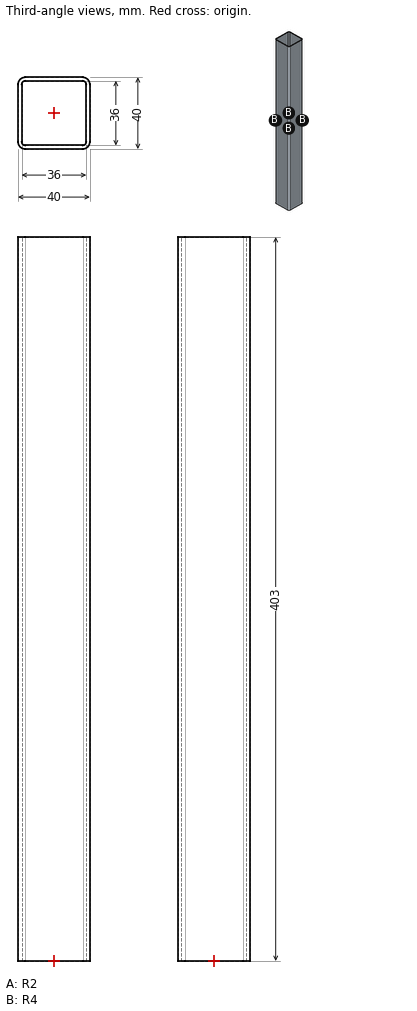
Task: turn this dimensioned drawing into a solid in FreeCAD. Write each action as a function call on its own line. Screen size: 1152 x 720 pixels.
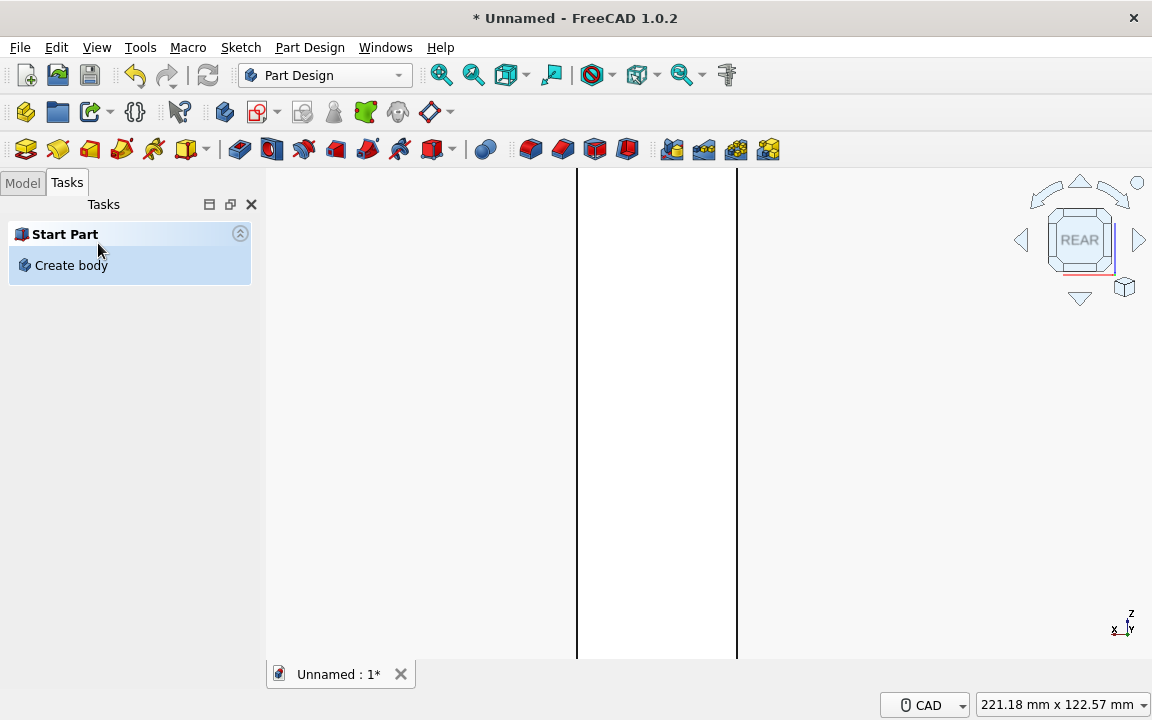
key(v)
key(f)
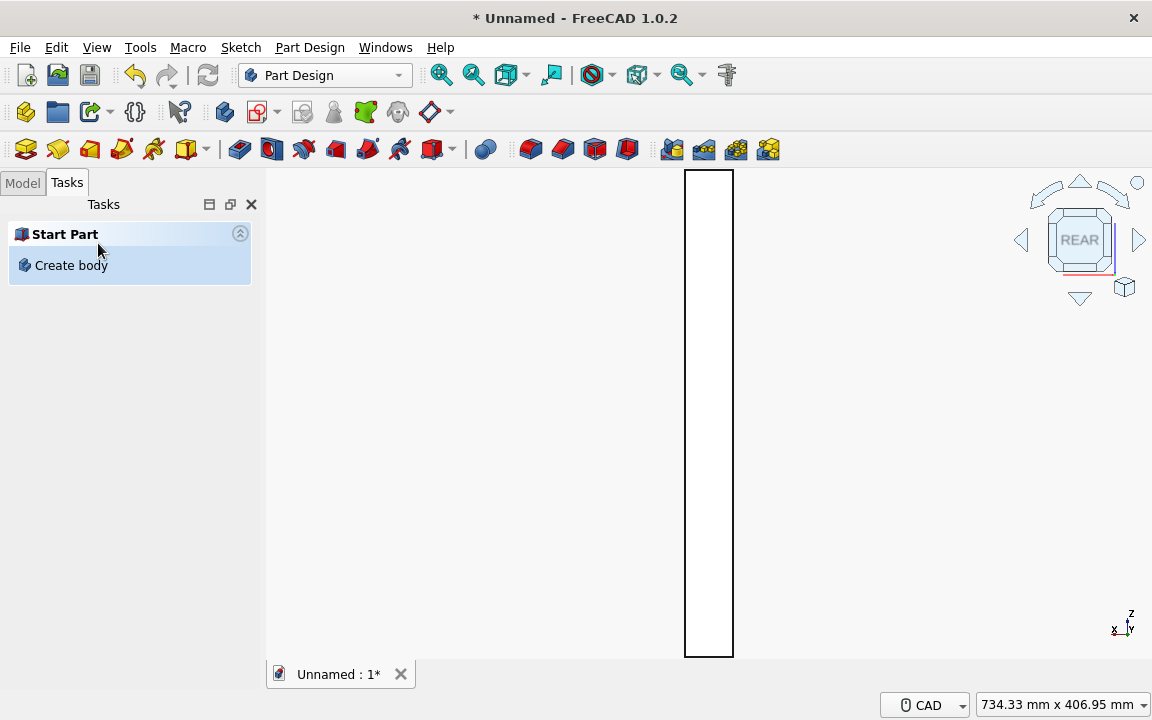
click(733, 413)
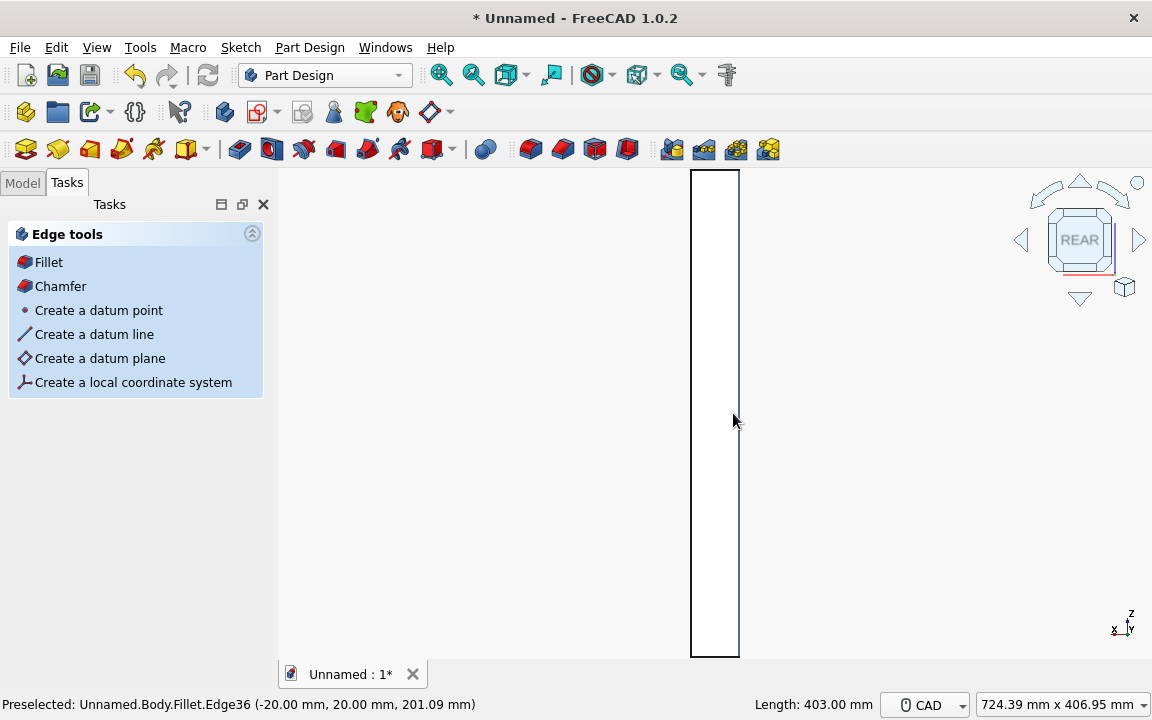
click(691, 413, ctrl)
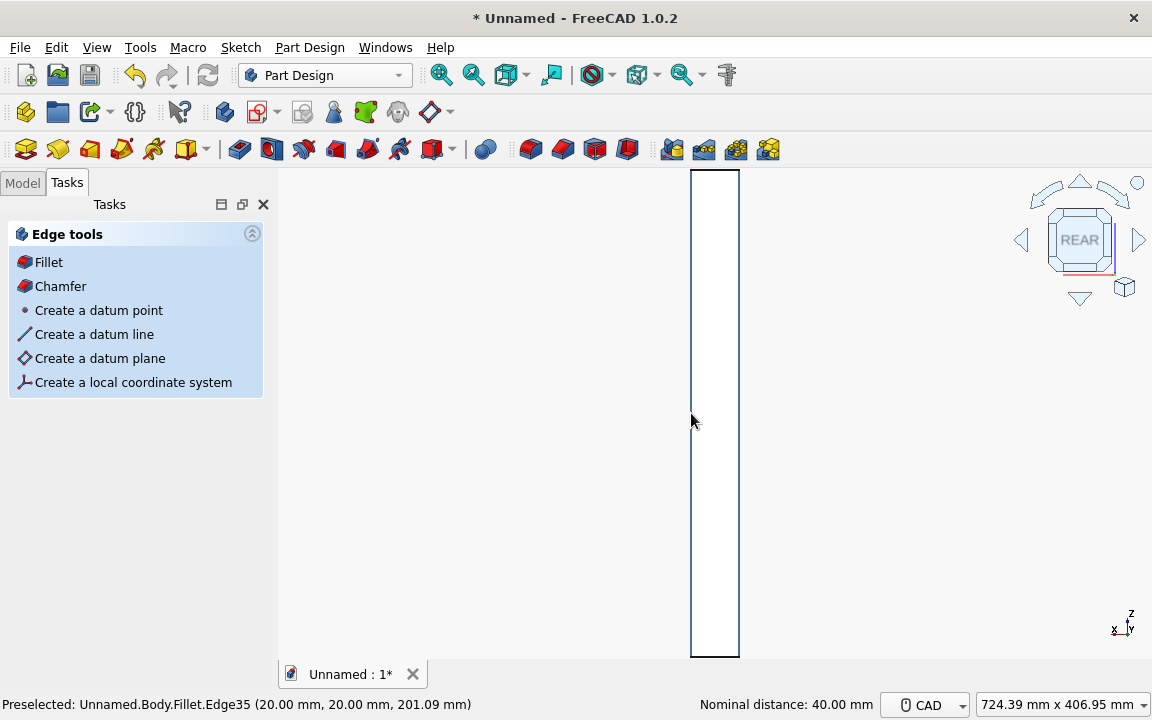
key(0)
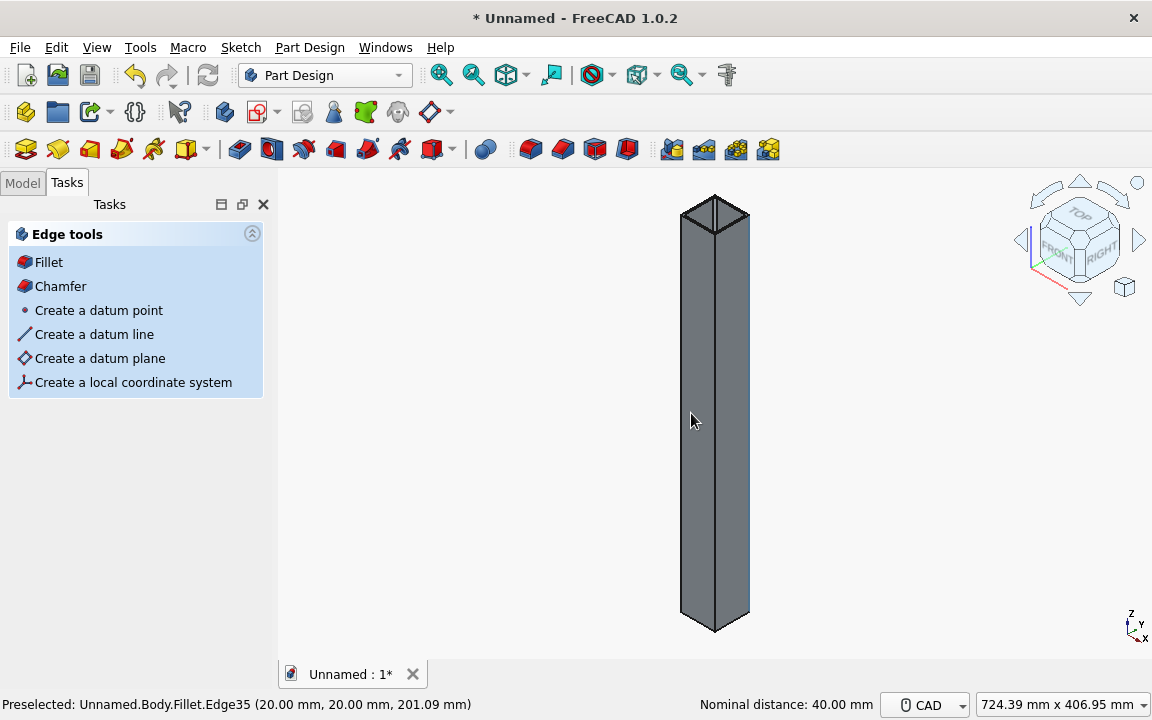
click(715, 432, ctrl)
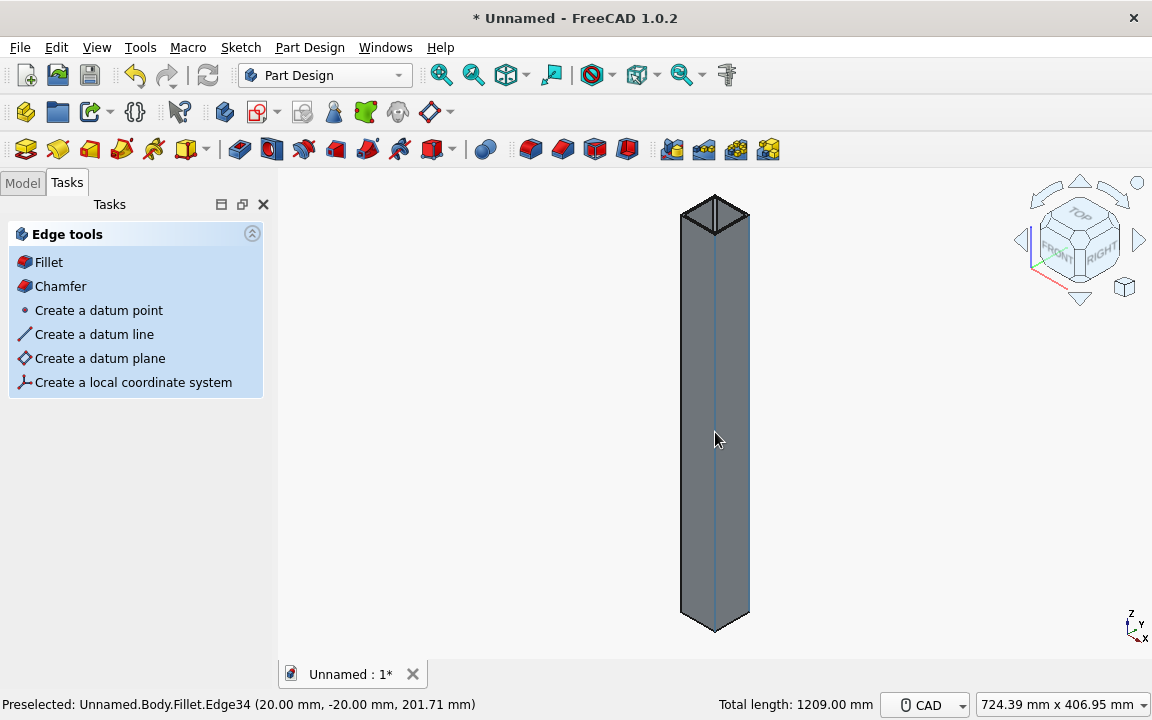
key(2)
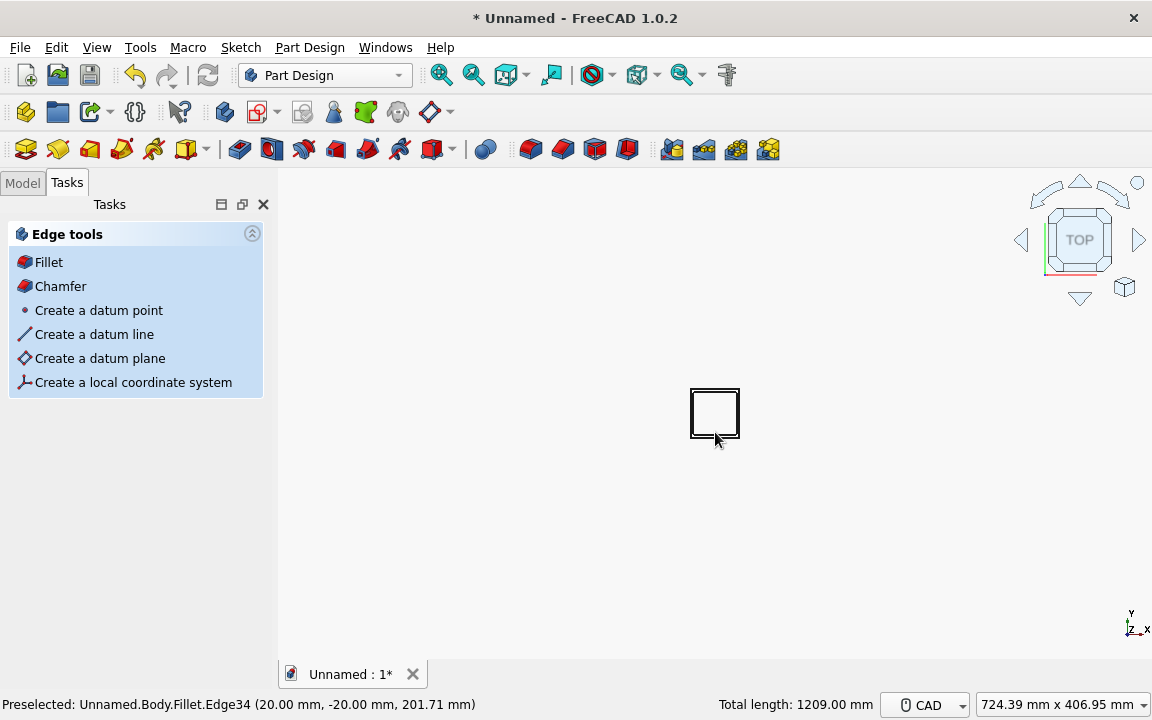
key(v)
key(f)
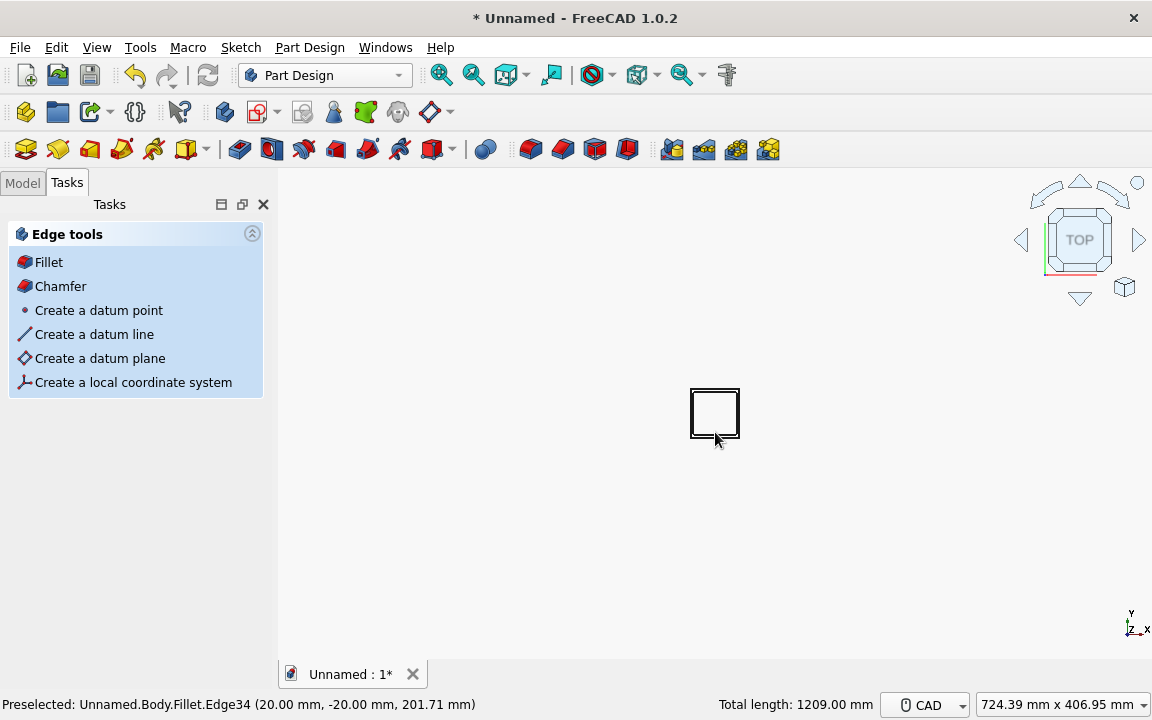
key(1)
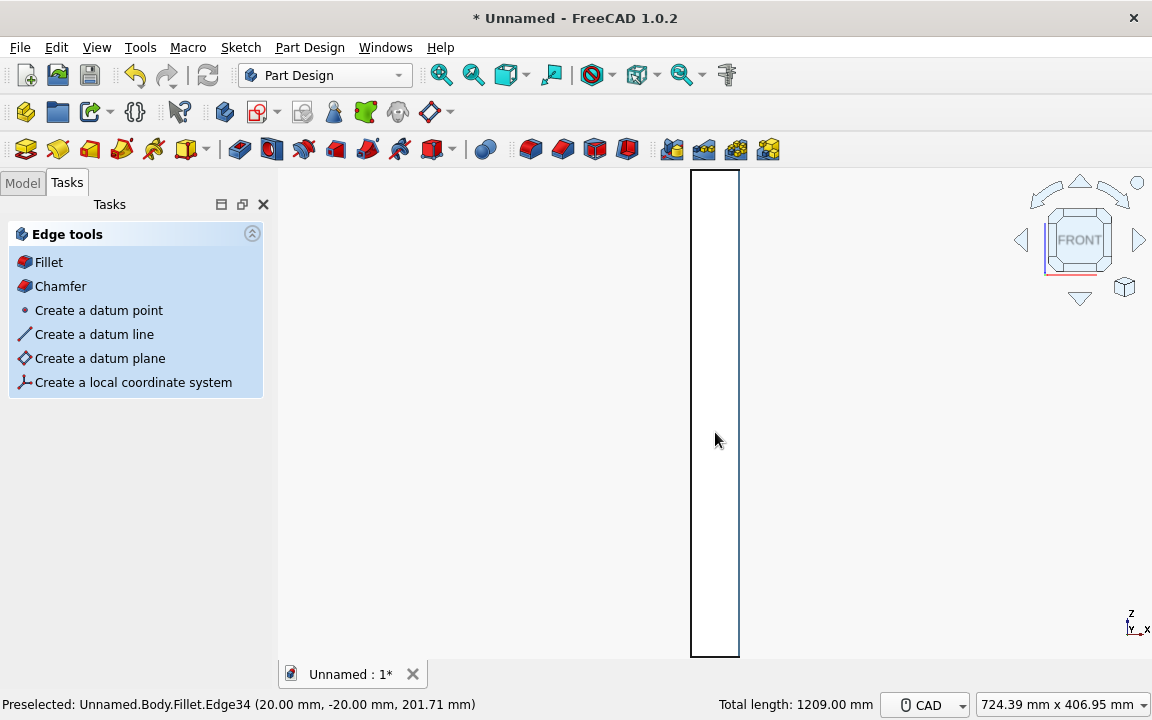
click(691, 412, ctrl)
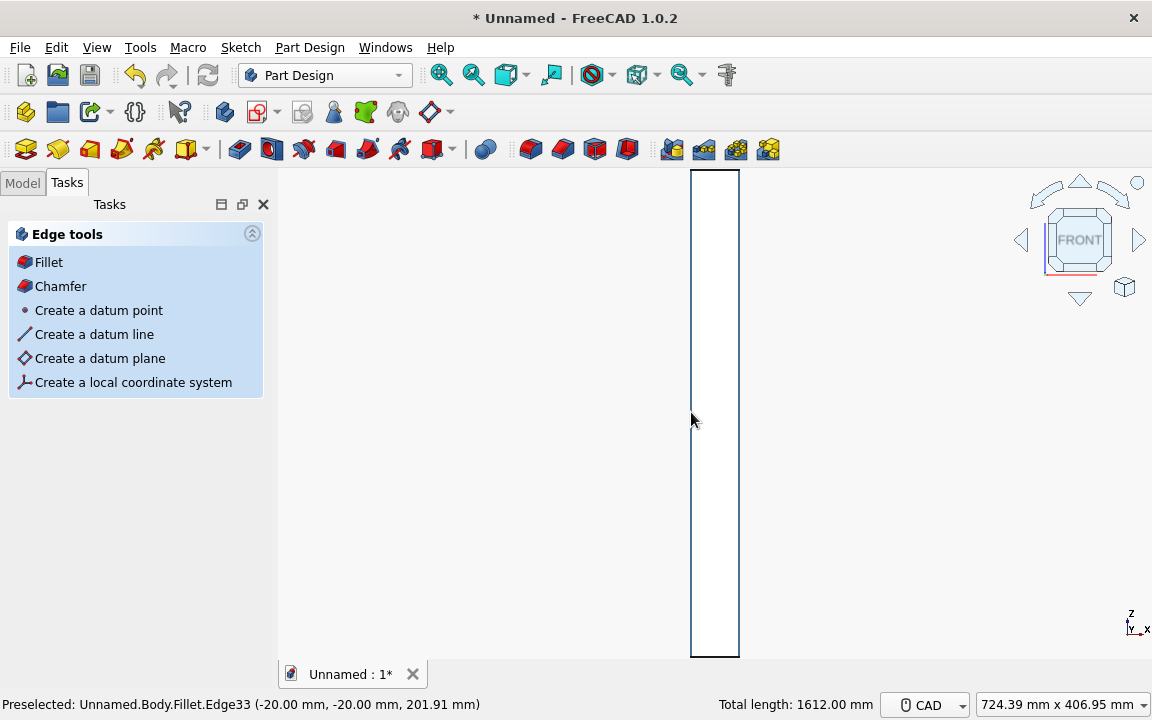
click(532, 150)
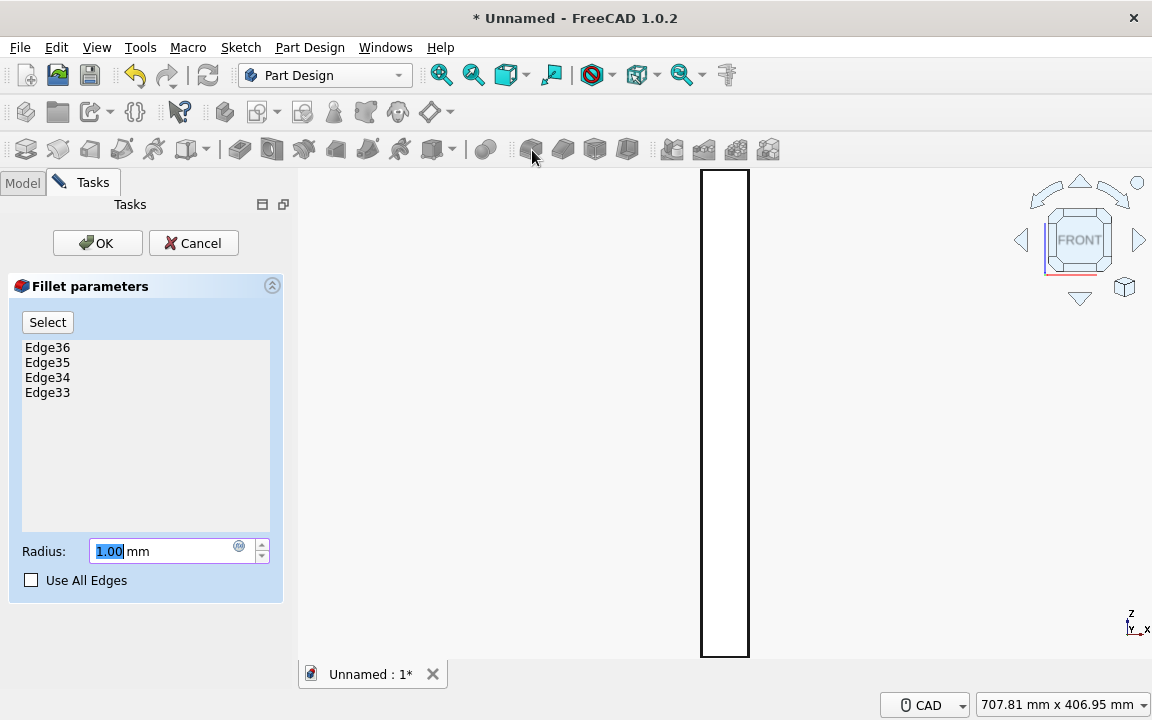
text(4)
key(Tab)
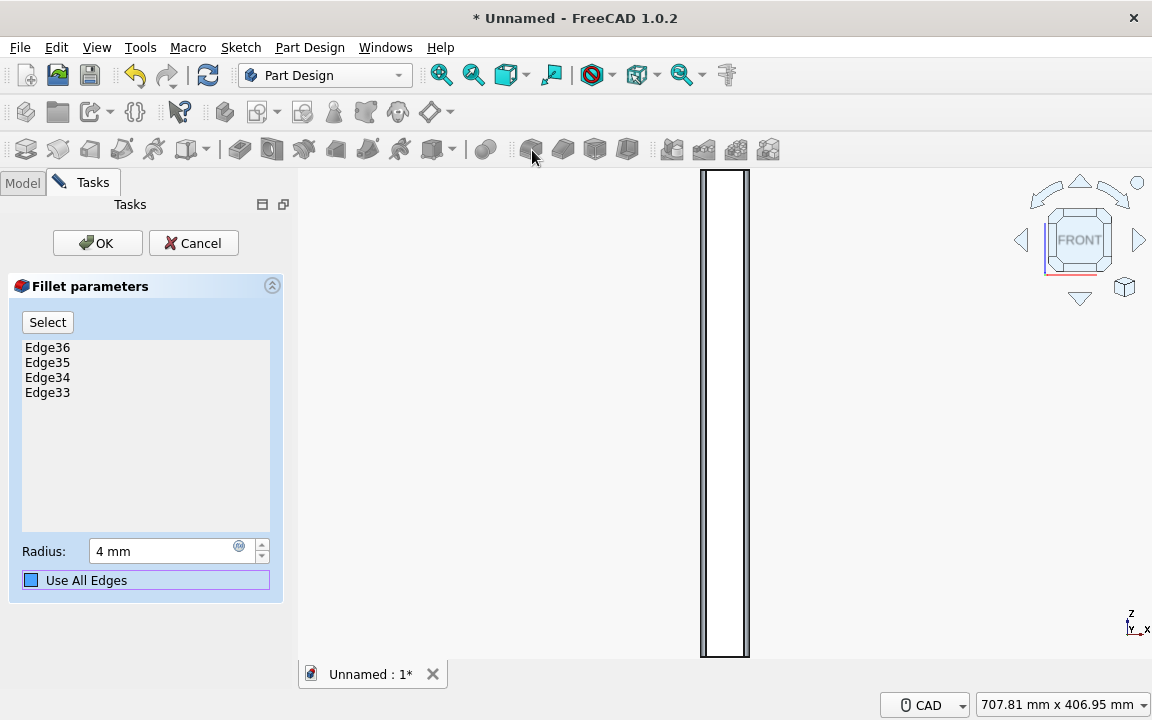
click(98, 243)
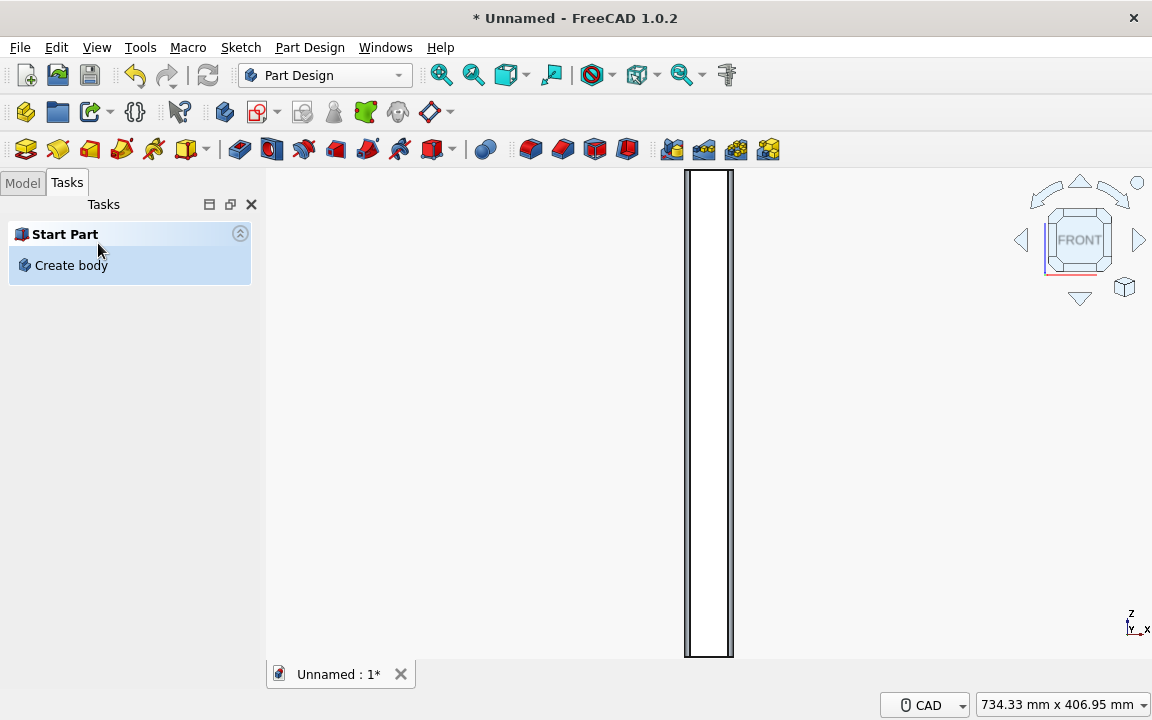
key(0)